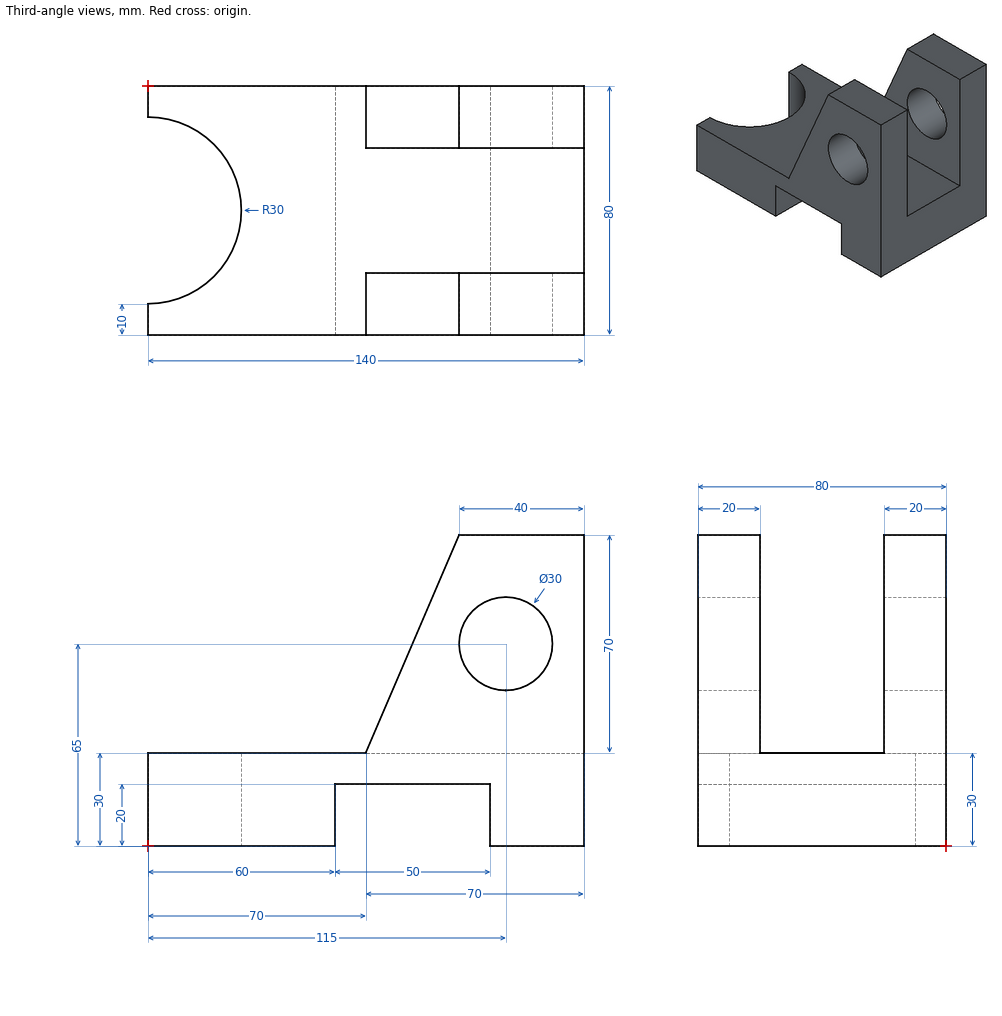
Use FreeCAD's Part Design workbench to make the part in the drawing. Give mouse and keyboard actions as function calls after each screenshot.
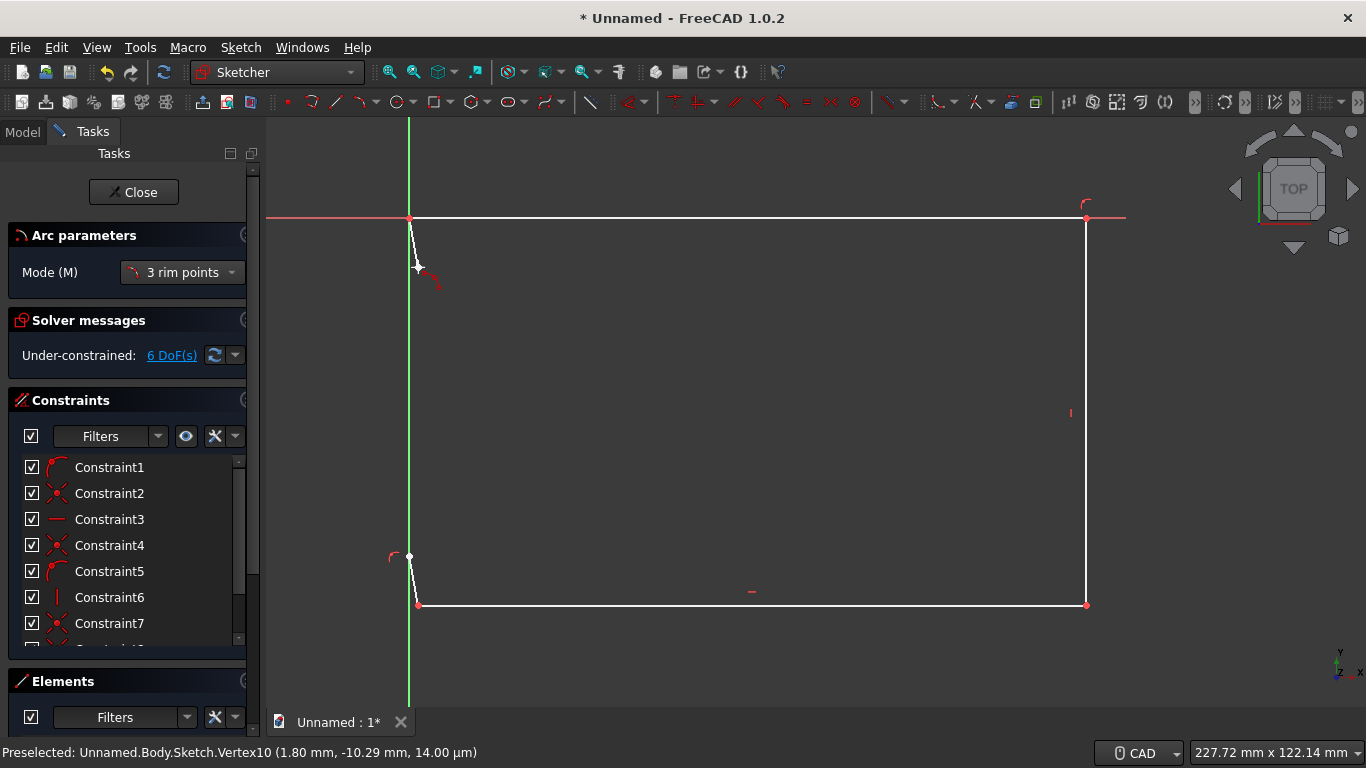
click(418, 268)
click(409, 557)
click(554, 411)
key(Escape)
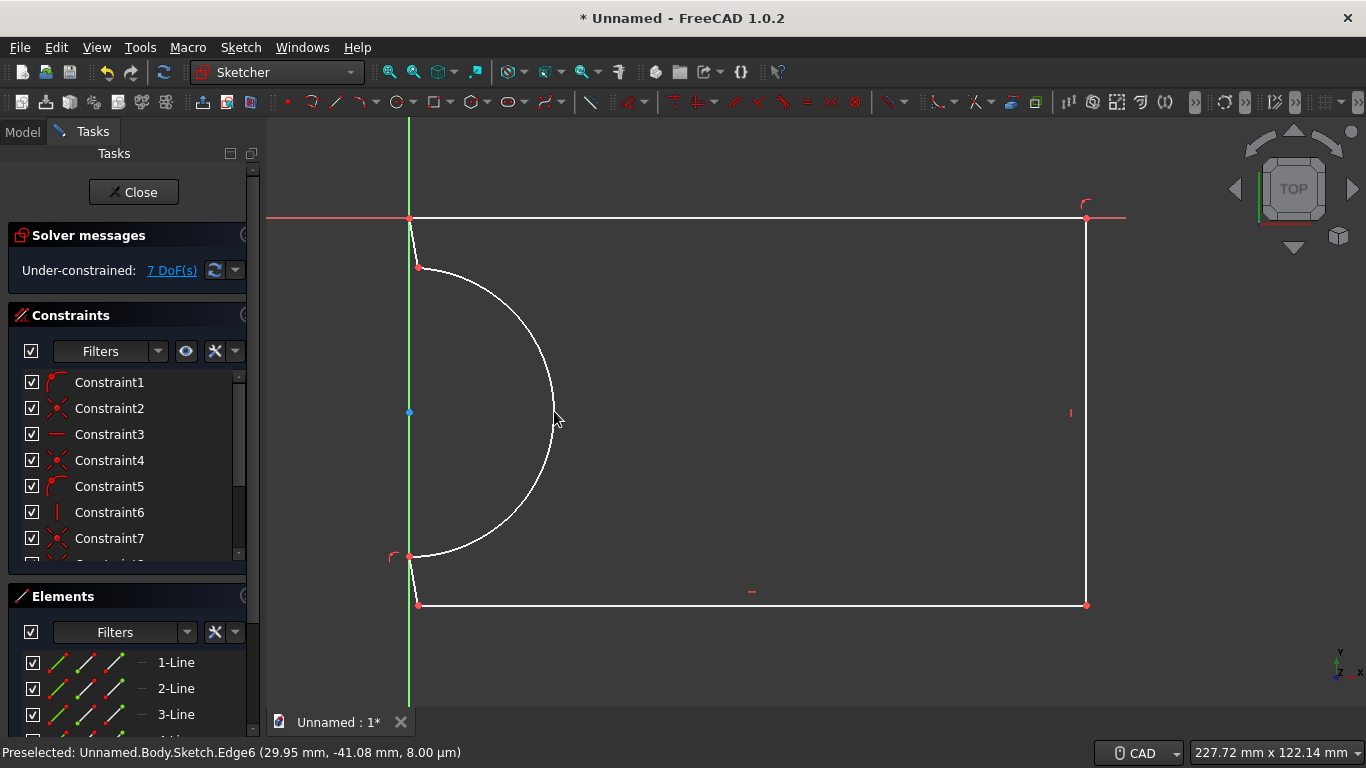
click(412, 572)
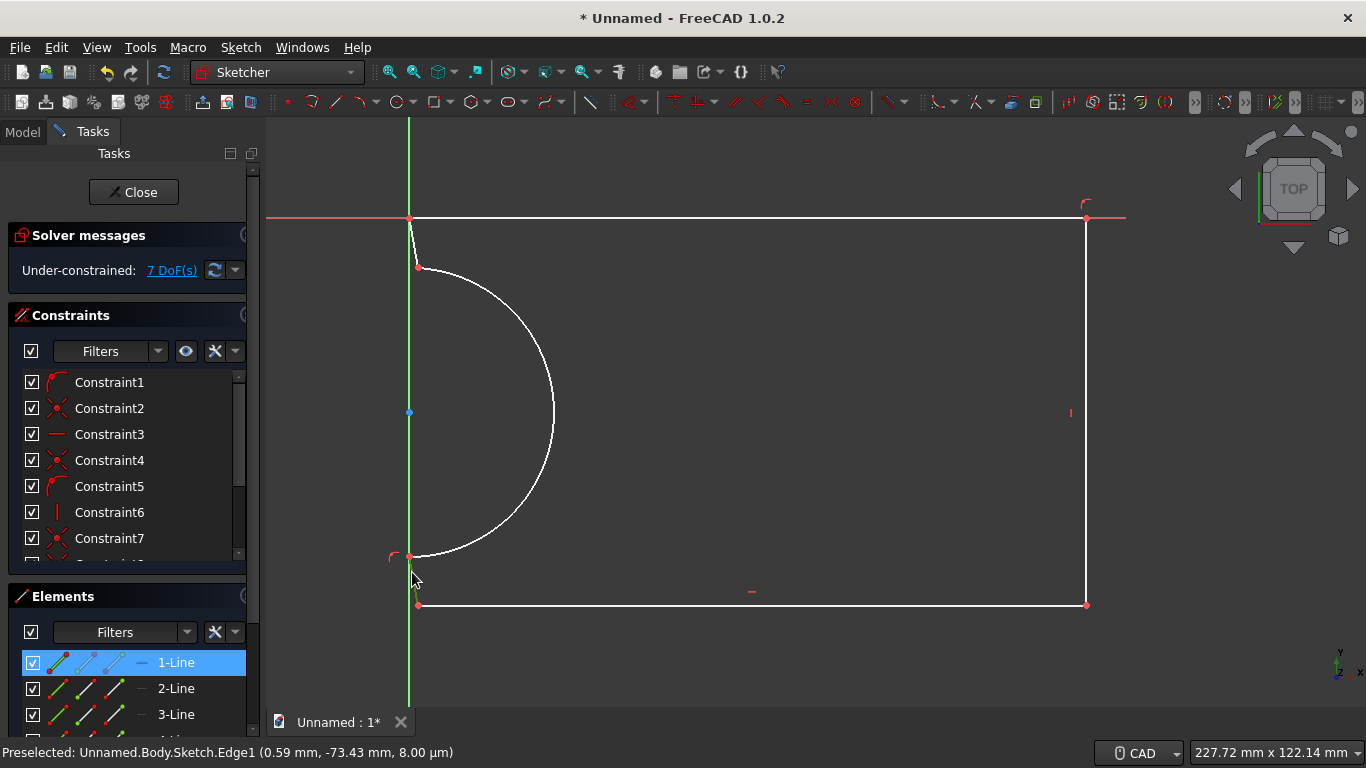
key(v)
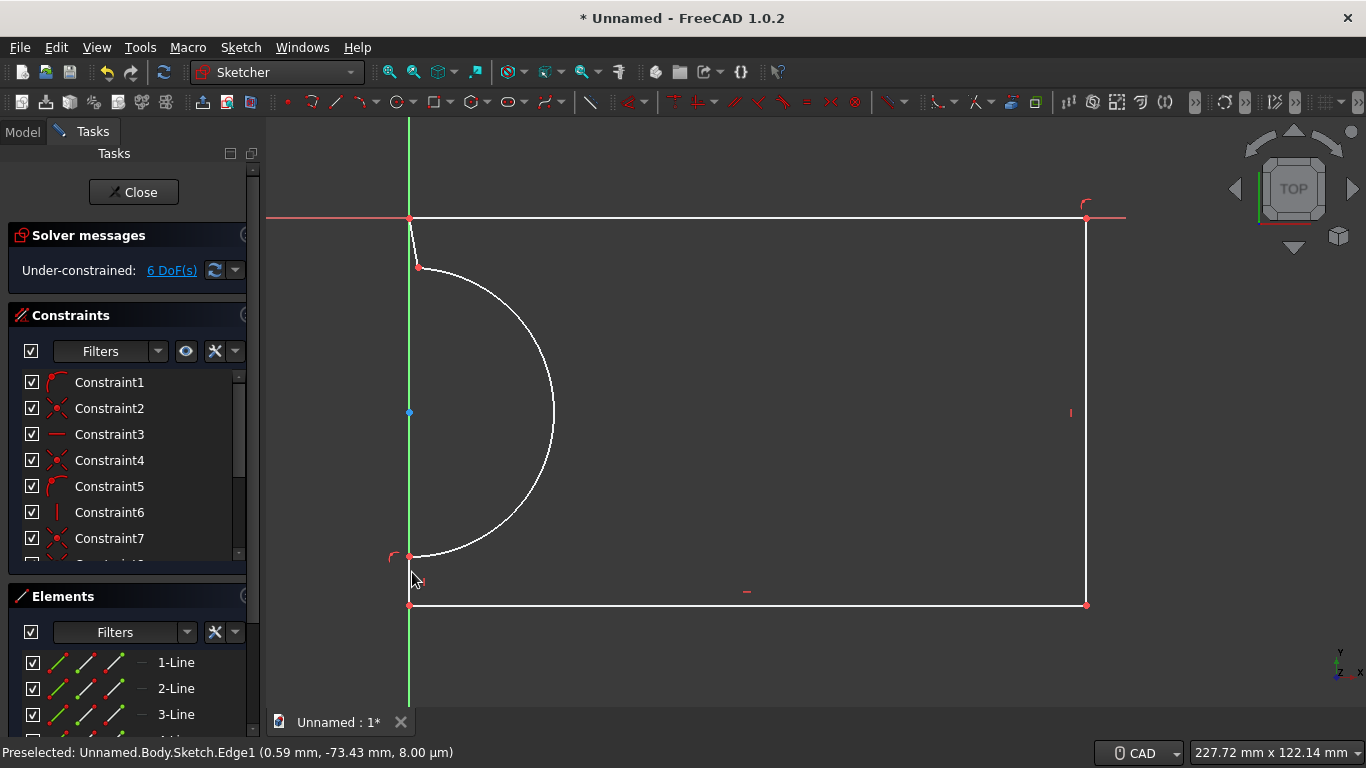
click(412, 233)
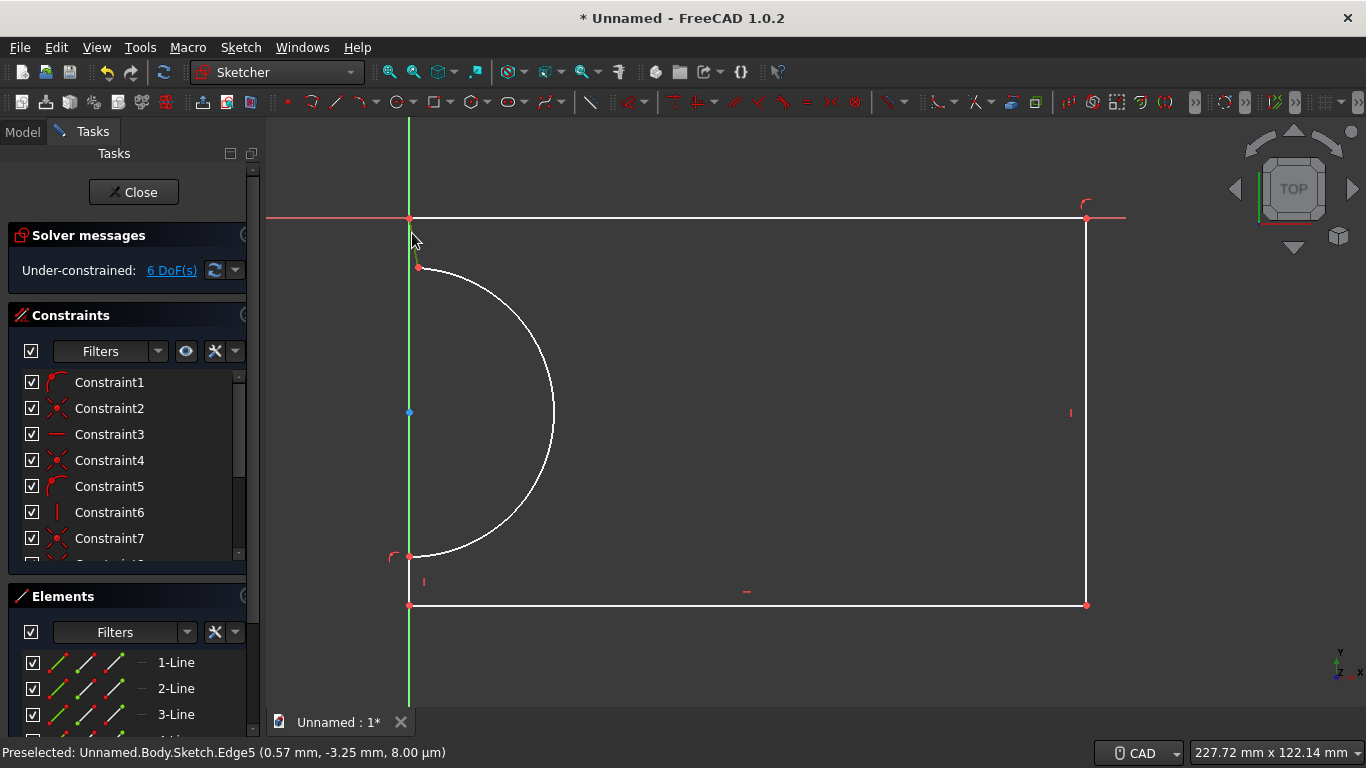
click(716, 102)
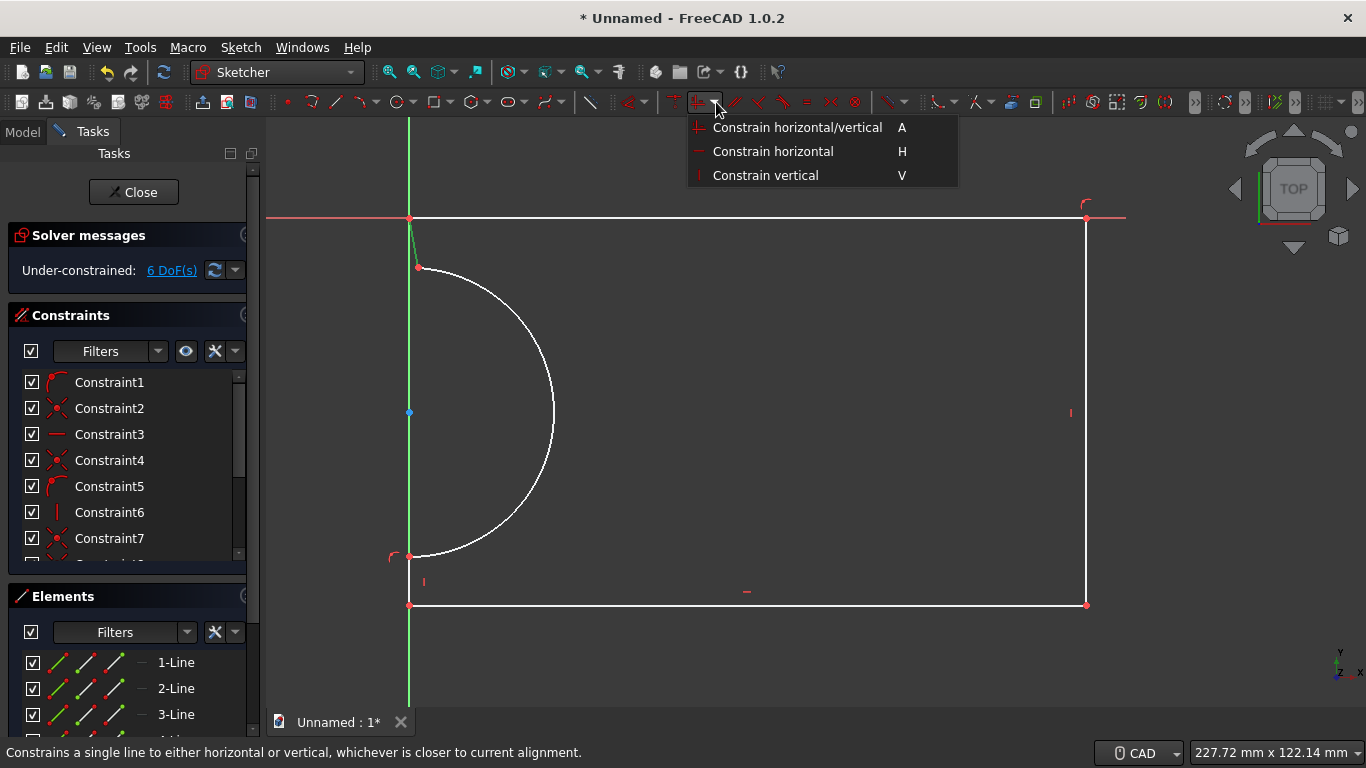
click(823, 175)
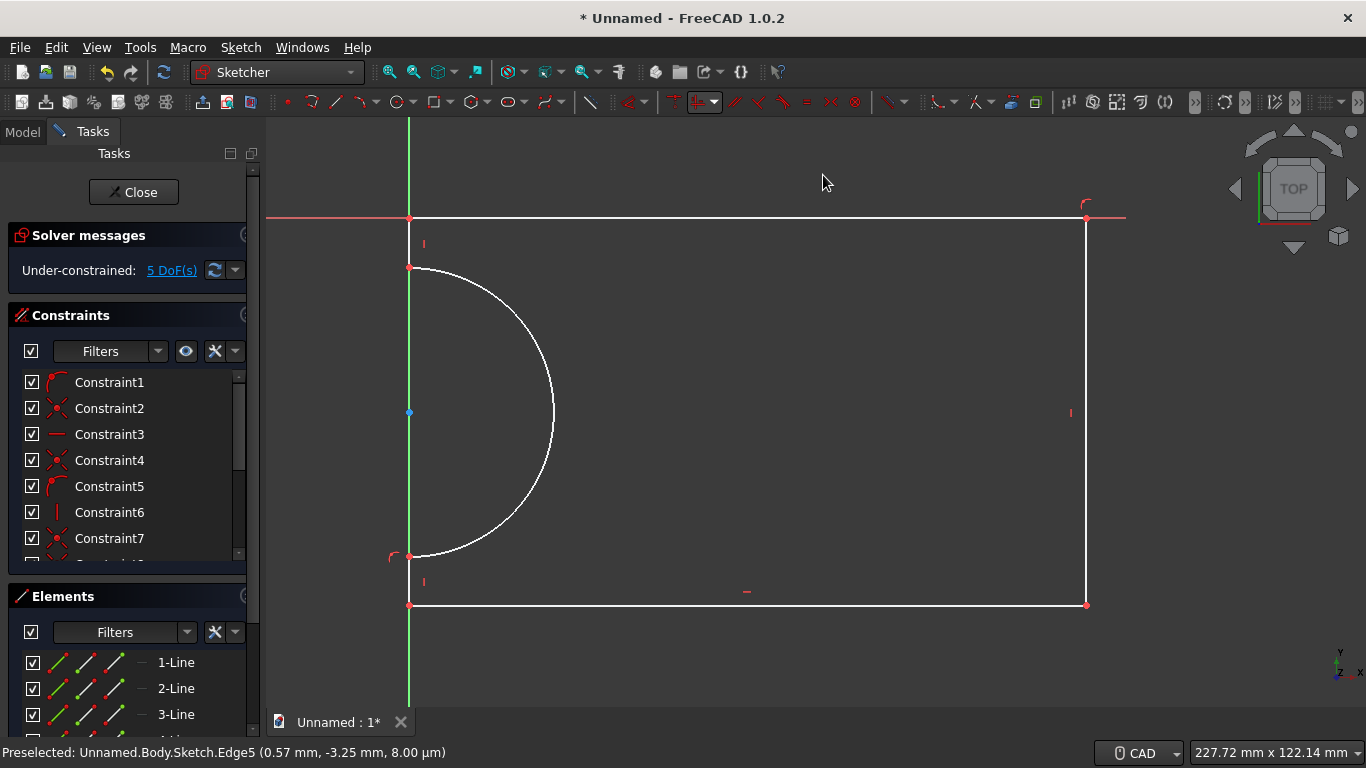
click(409, 412)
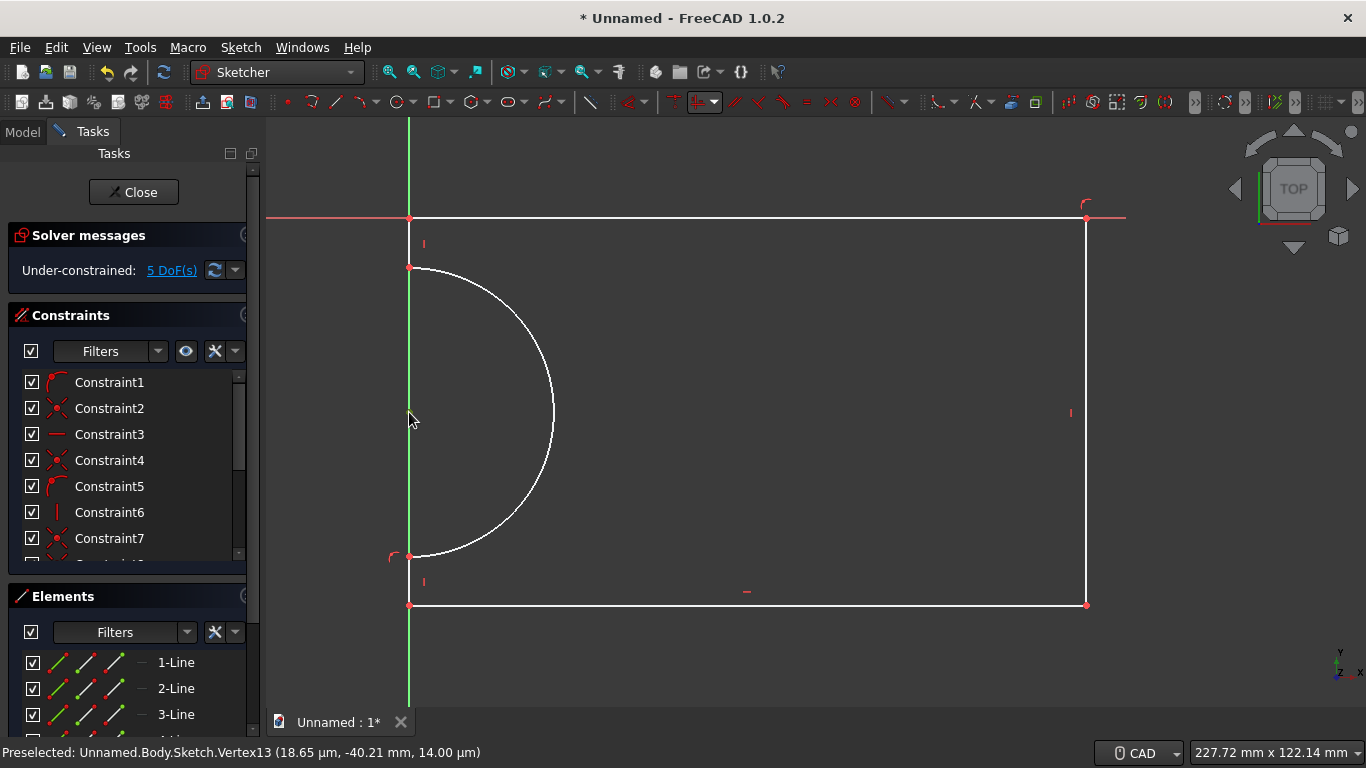
click(409, 641)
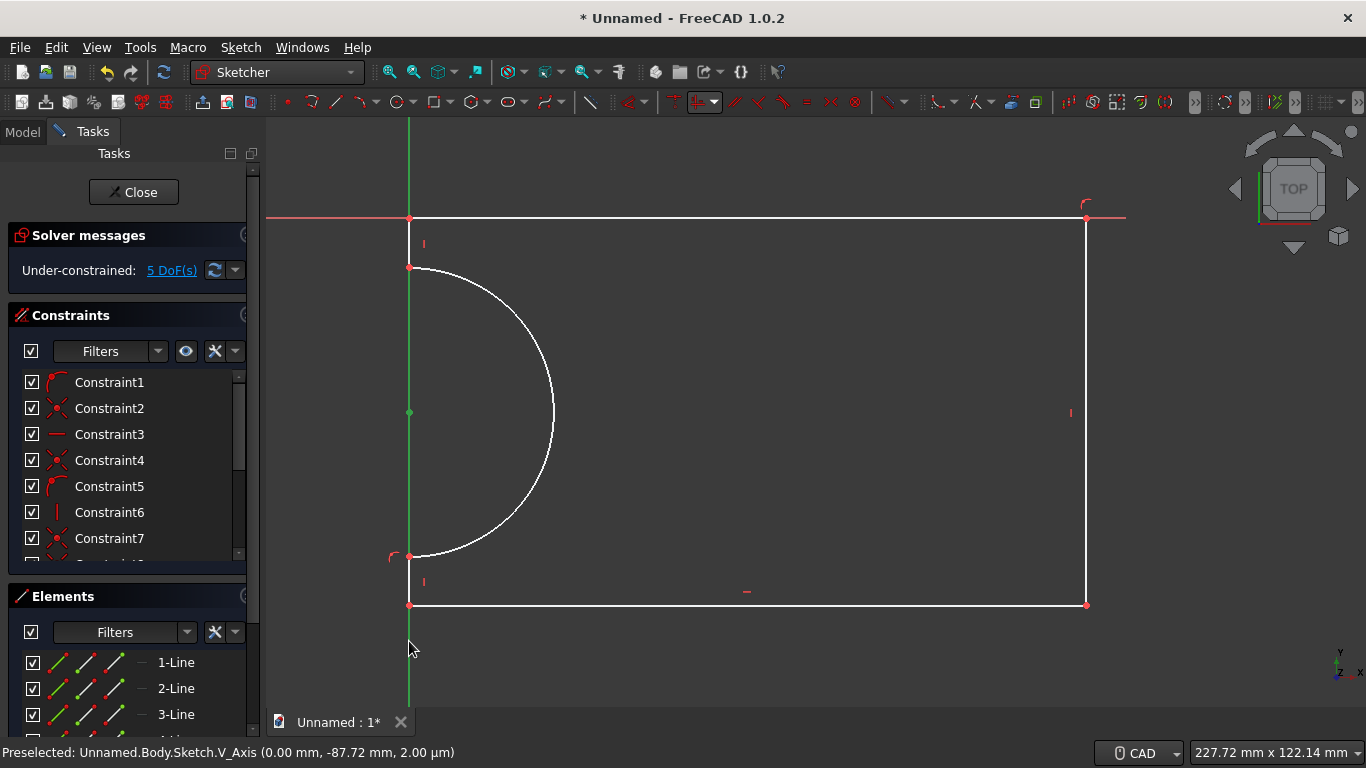
click(674, 102)